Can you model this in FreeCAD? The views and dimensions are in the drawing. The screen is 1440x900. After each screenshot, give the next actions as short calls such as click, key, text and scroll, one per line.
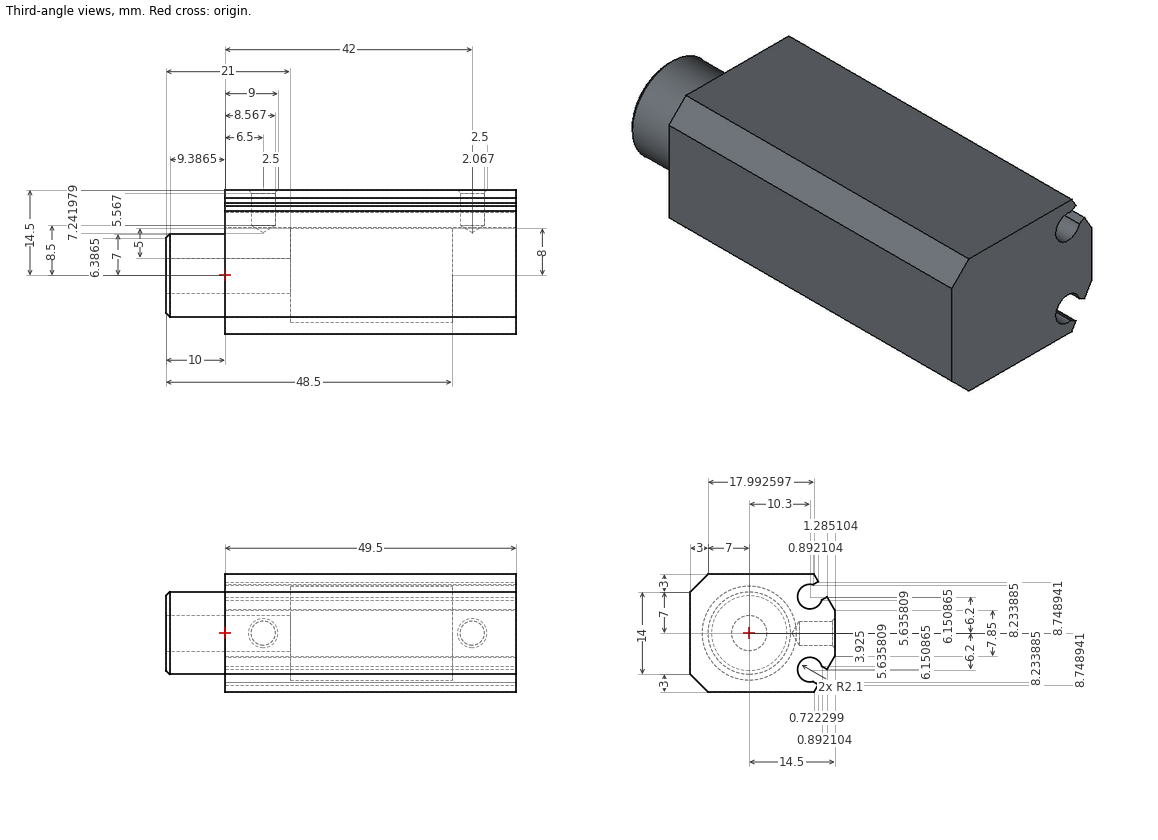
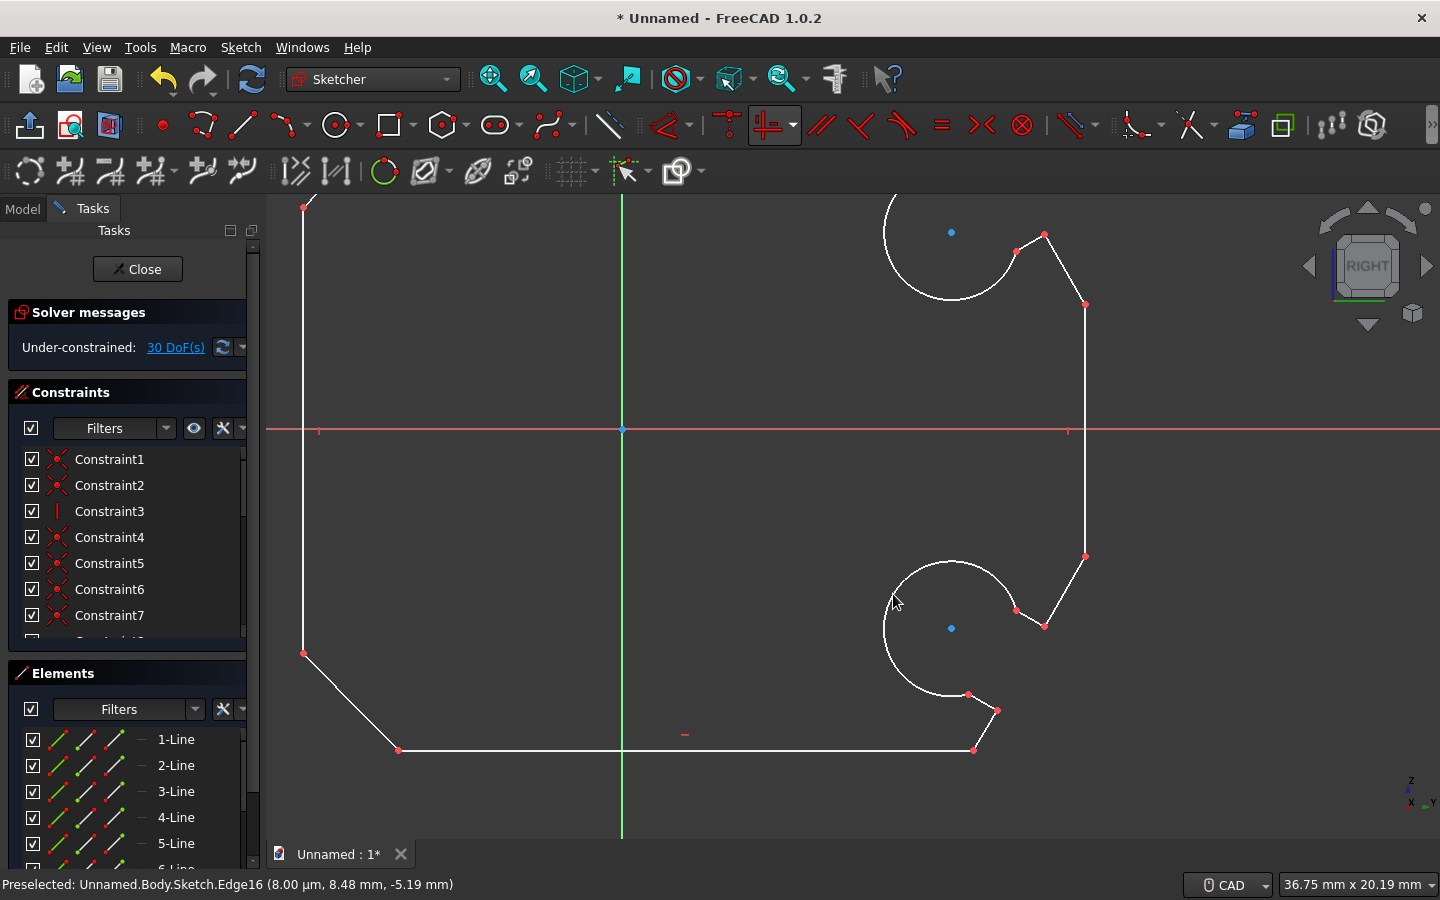
click(944, 300)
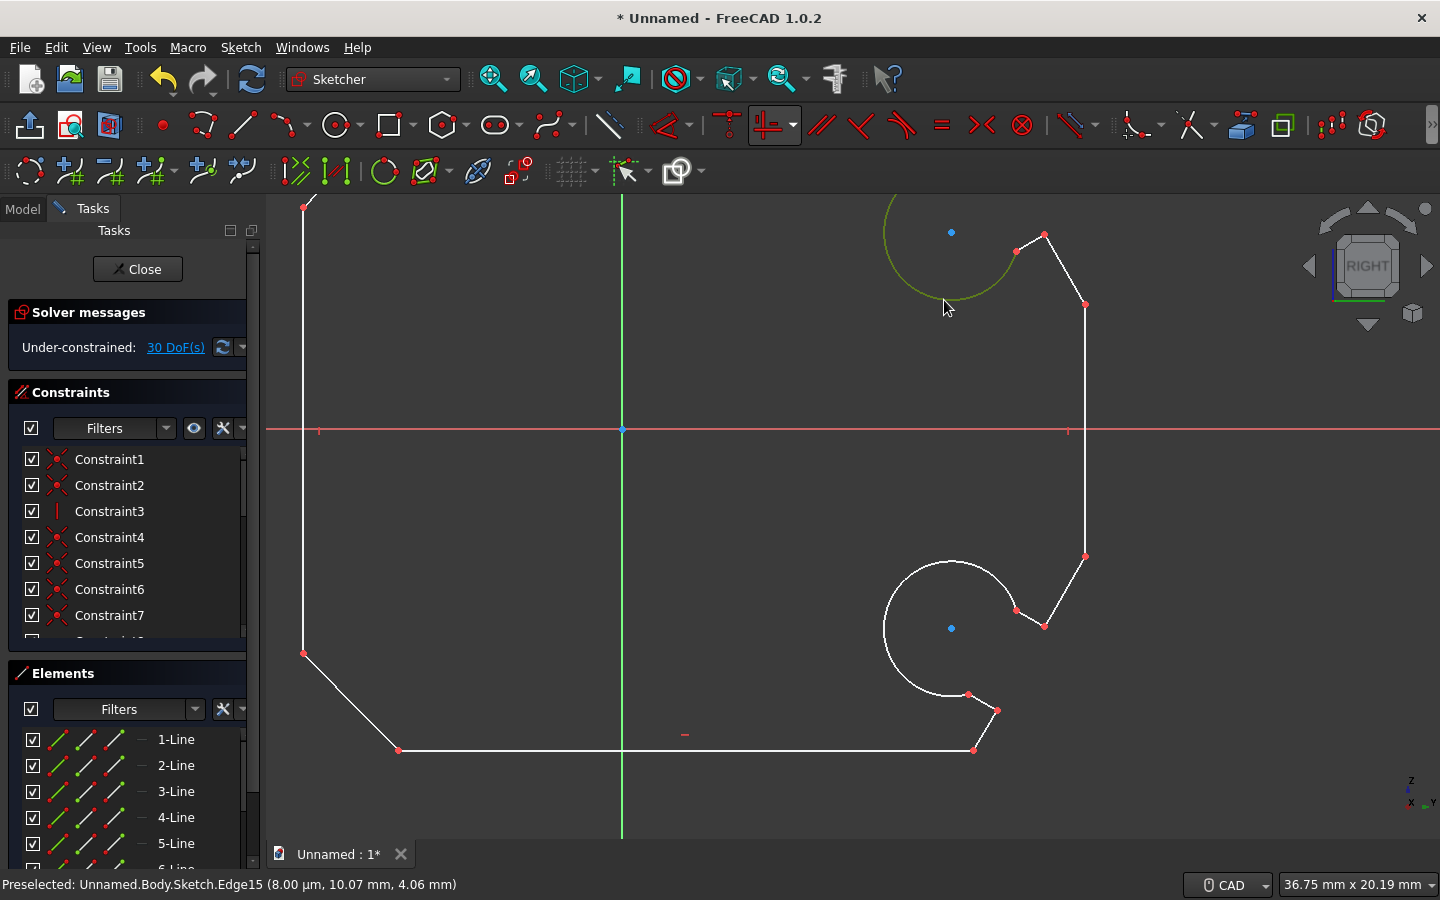
click(944, 562)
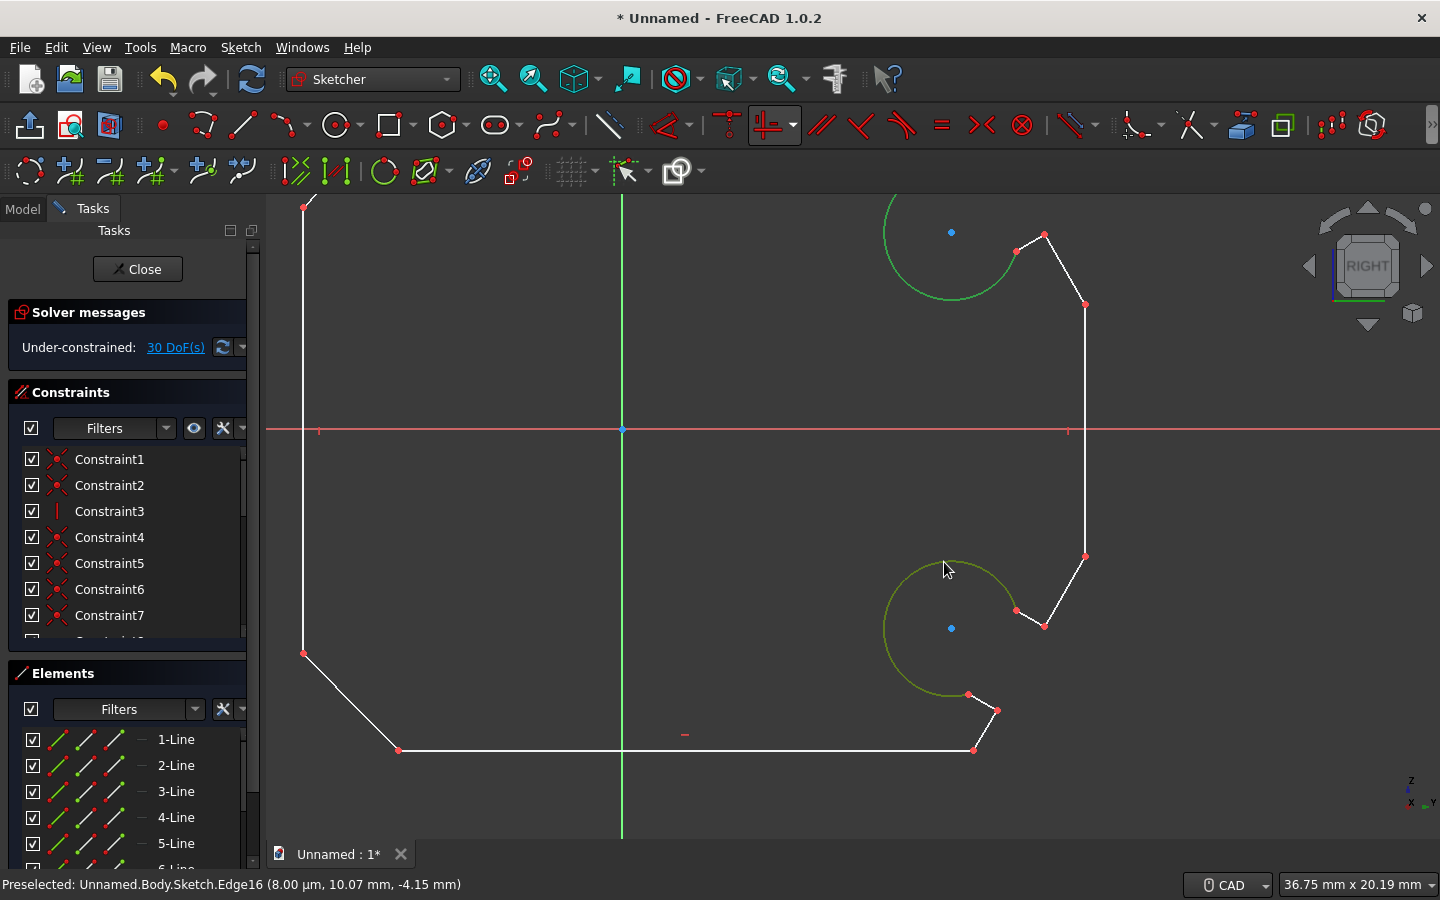
click(942, 126)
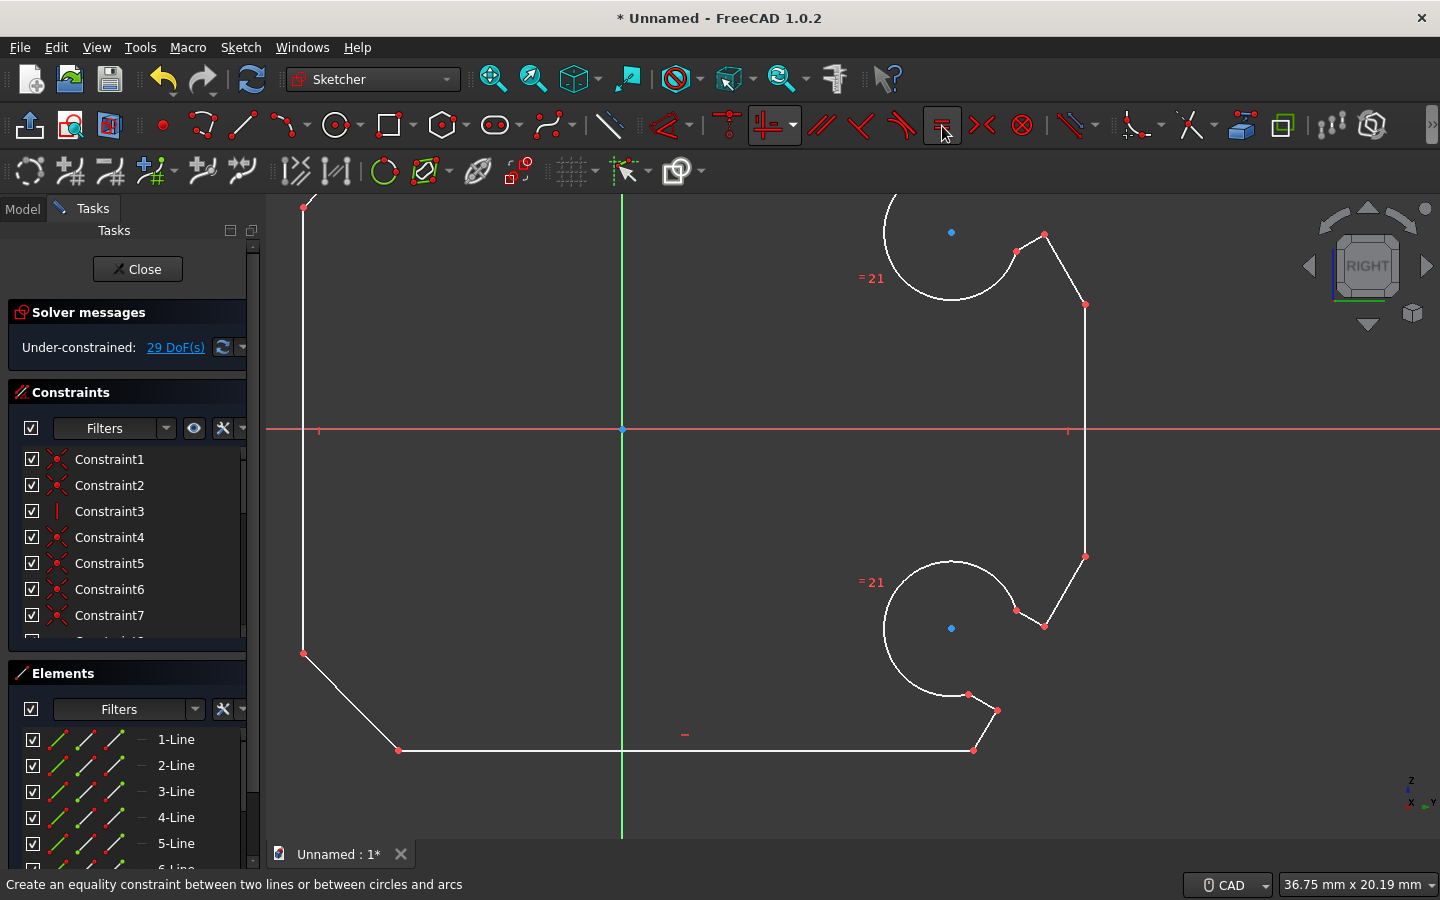
click(664, 126)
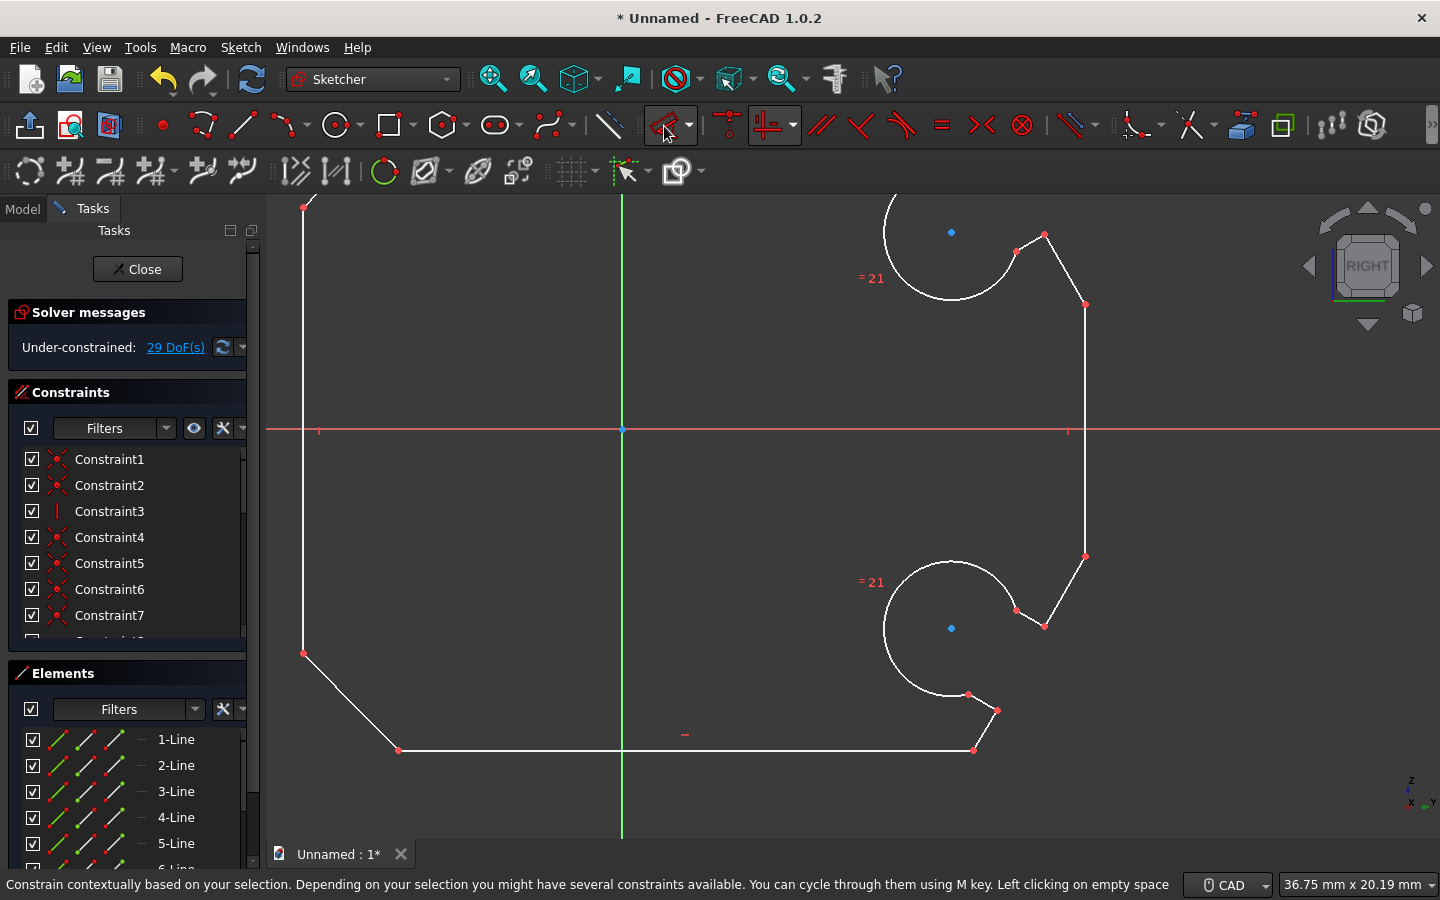
click(944, 300)
click(940, 332)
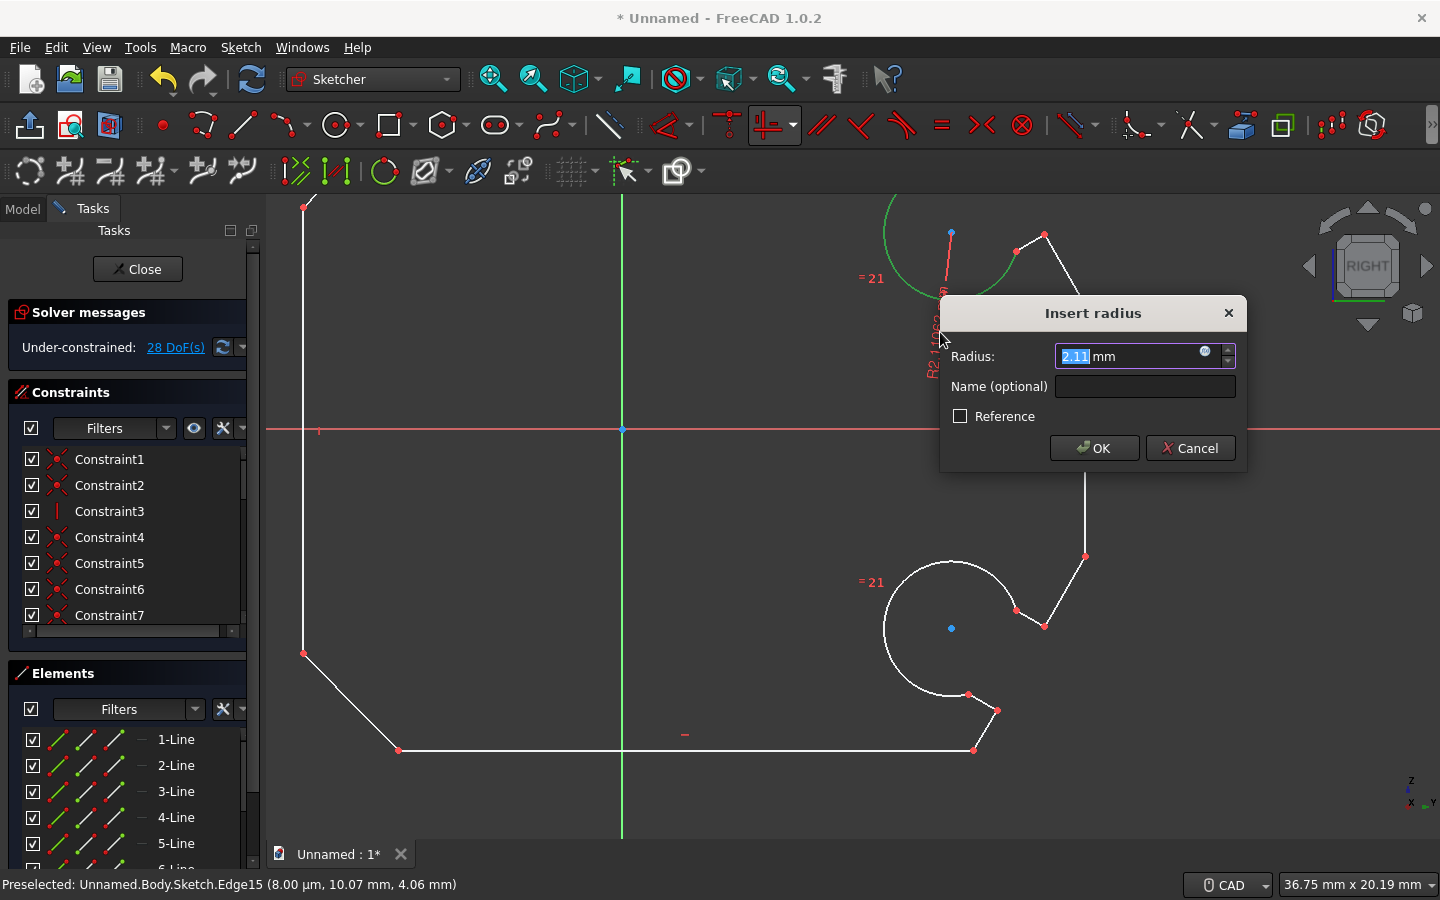
text(2.1)
key(Return)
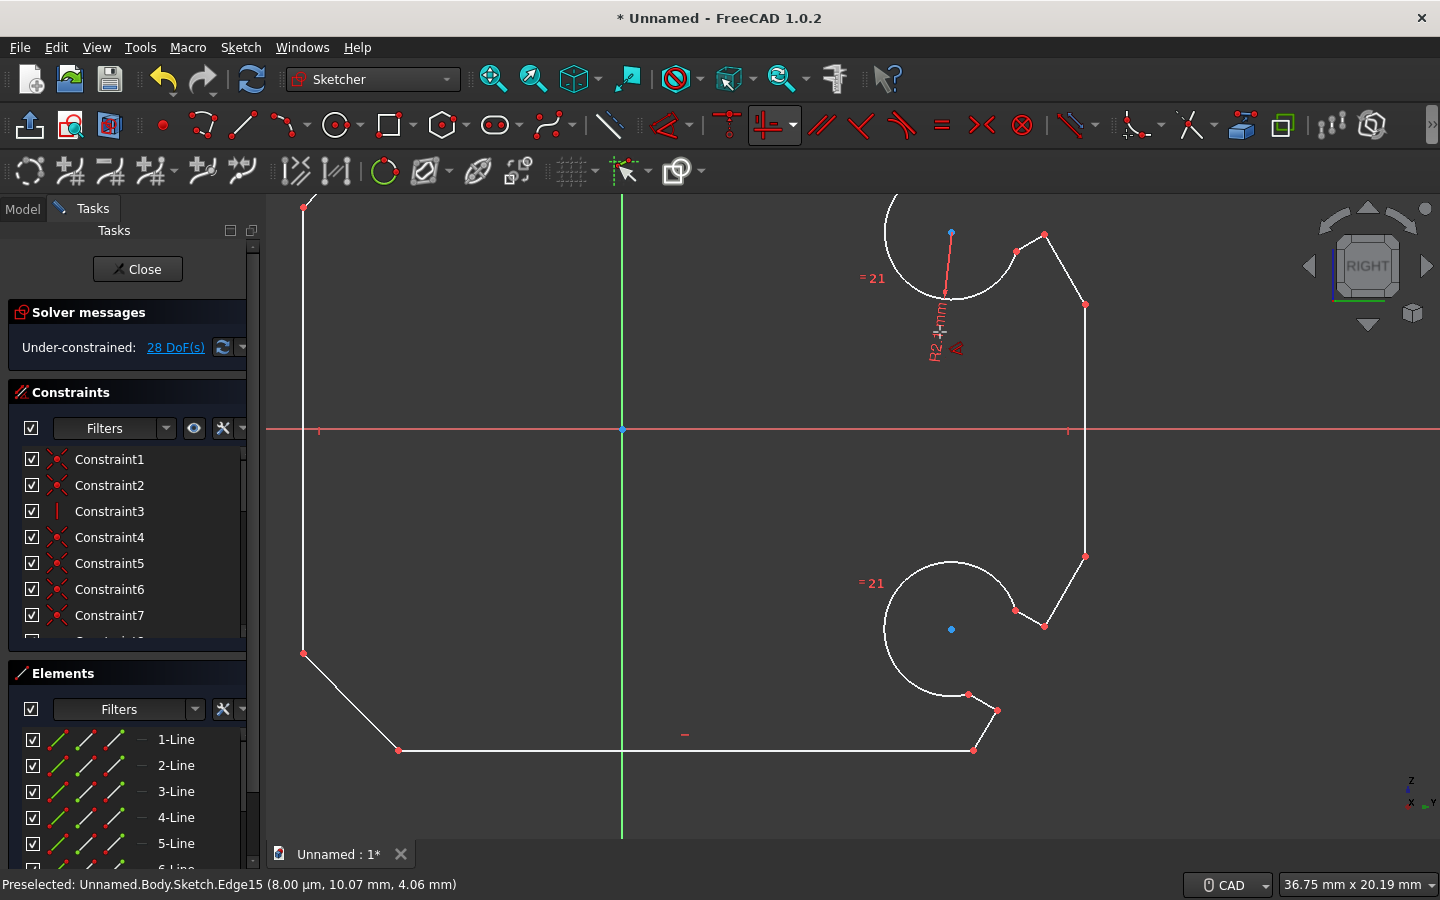
click(303, 342)
click(337, 339)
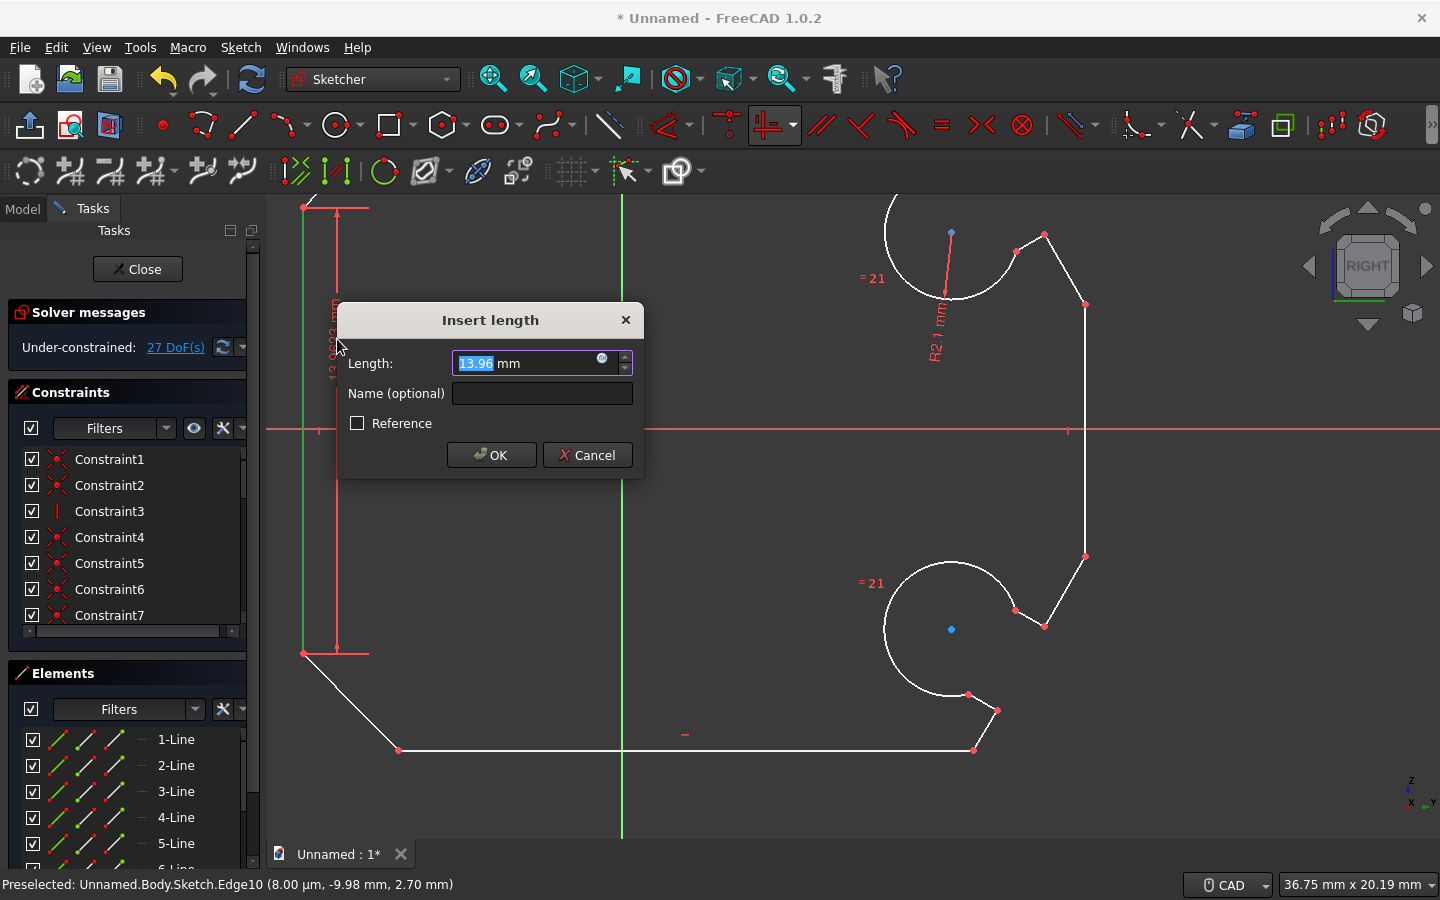
text(14)
key(Return)